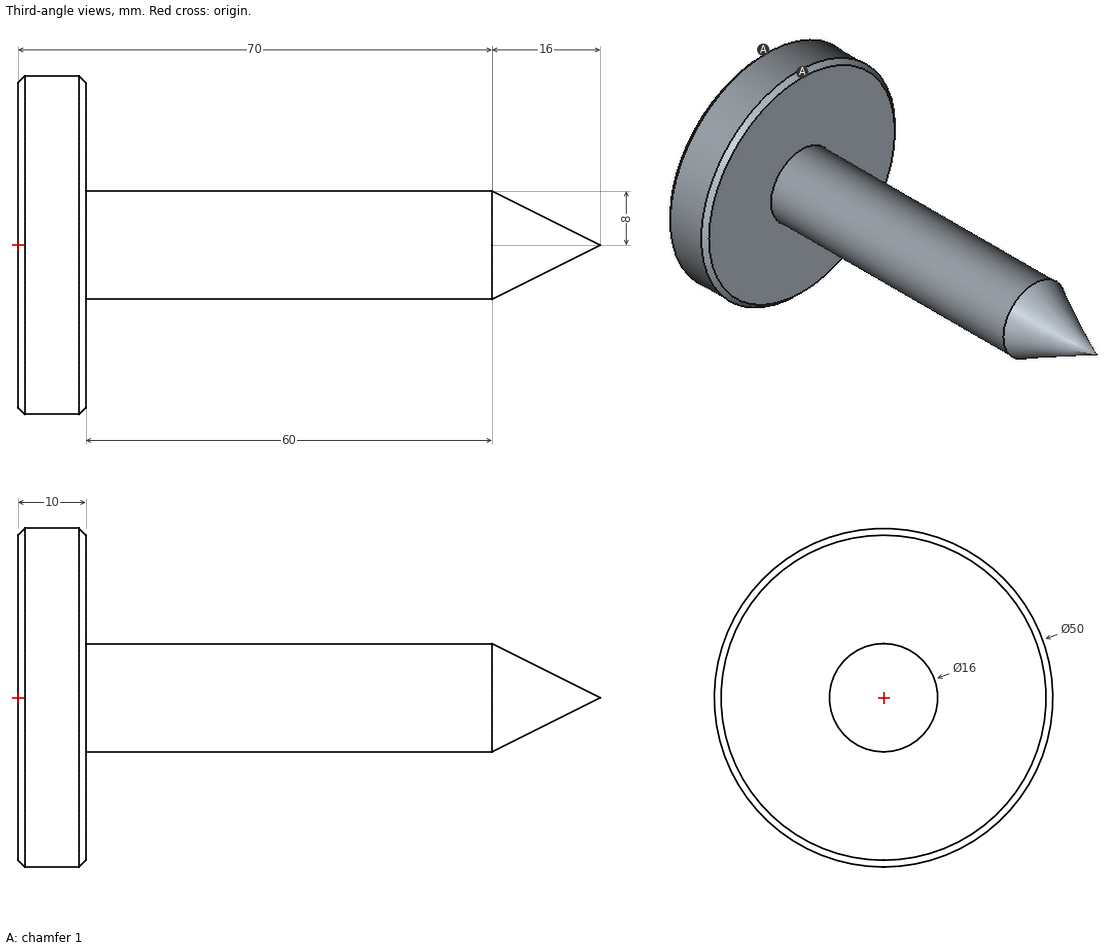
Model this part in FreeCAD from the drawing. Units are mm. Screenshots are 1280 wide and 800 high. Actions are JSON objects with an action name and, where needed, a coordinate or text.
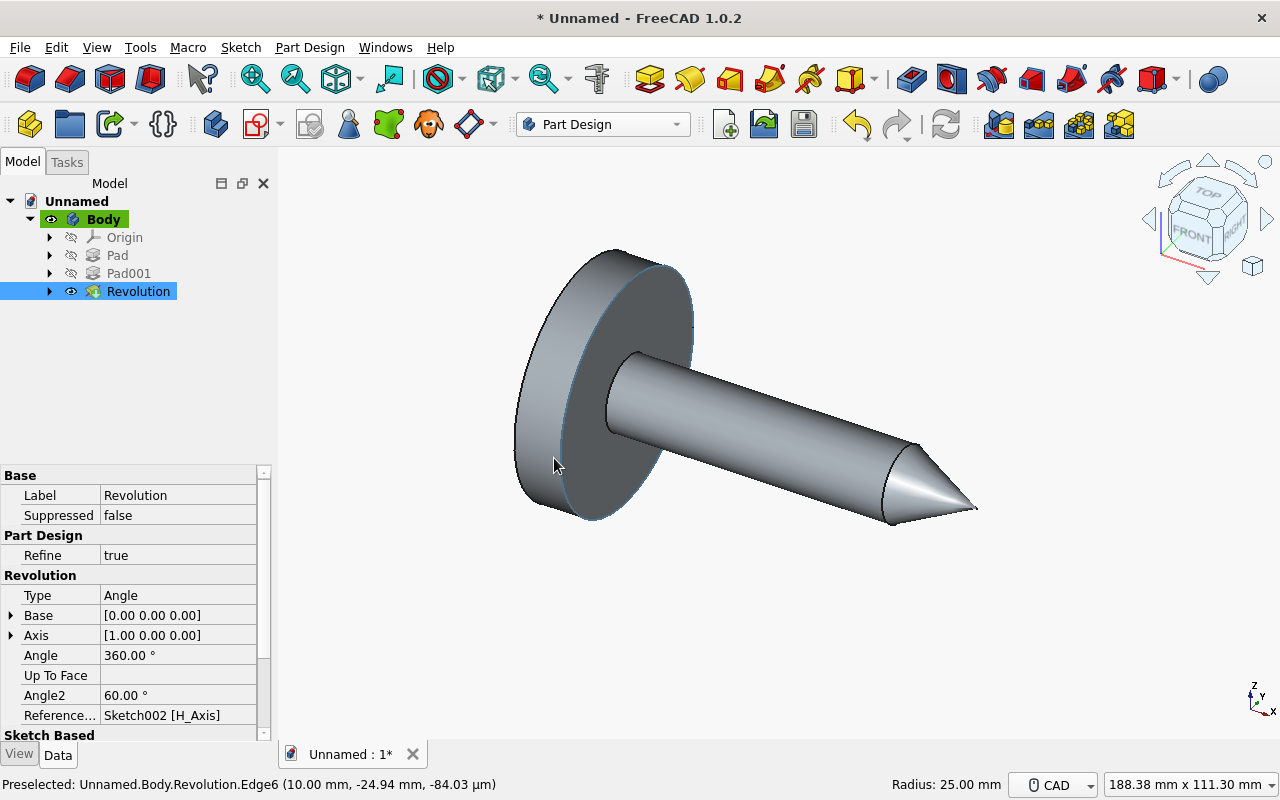
{"action": "key", "text": "0"}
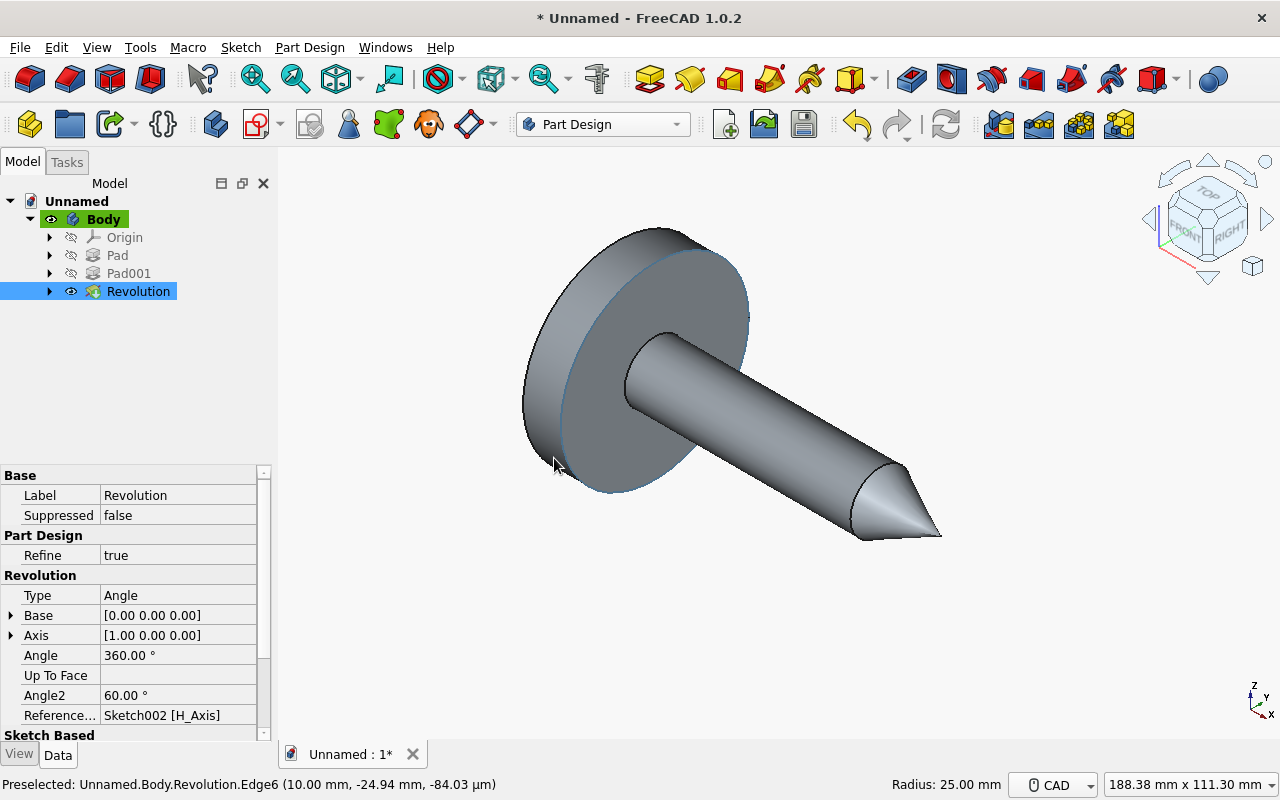
{"action": "key", "text": "2"}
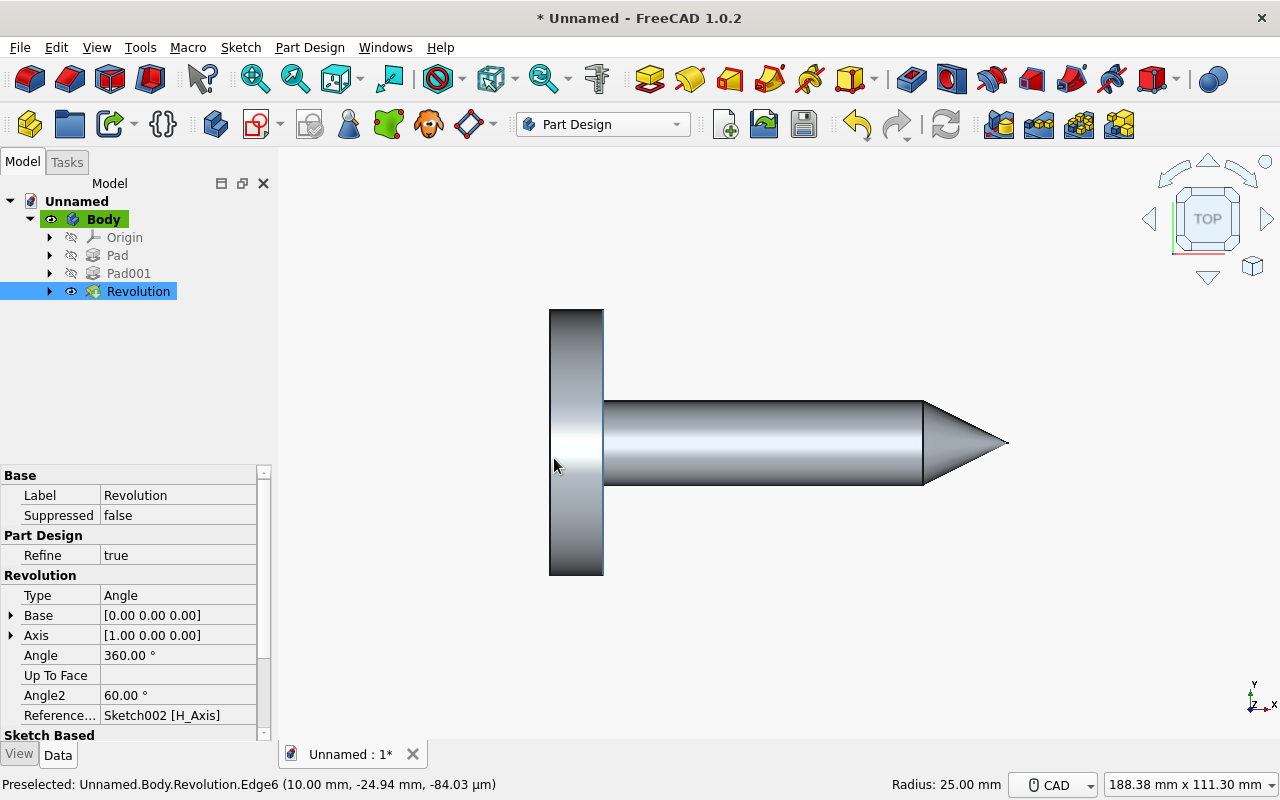
{"action": "left_click", "coordinate": [550, 550], "text": "ctrl"}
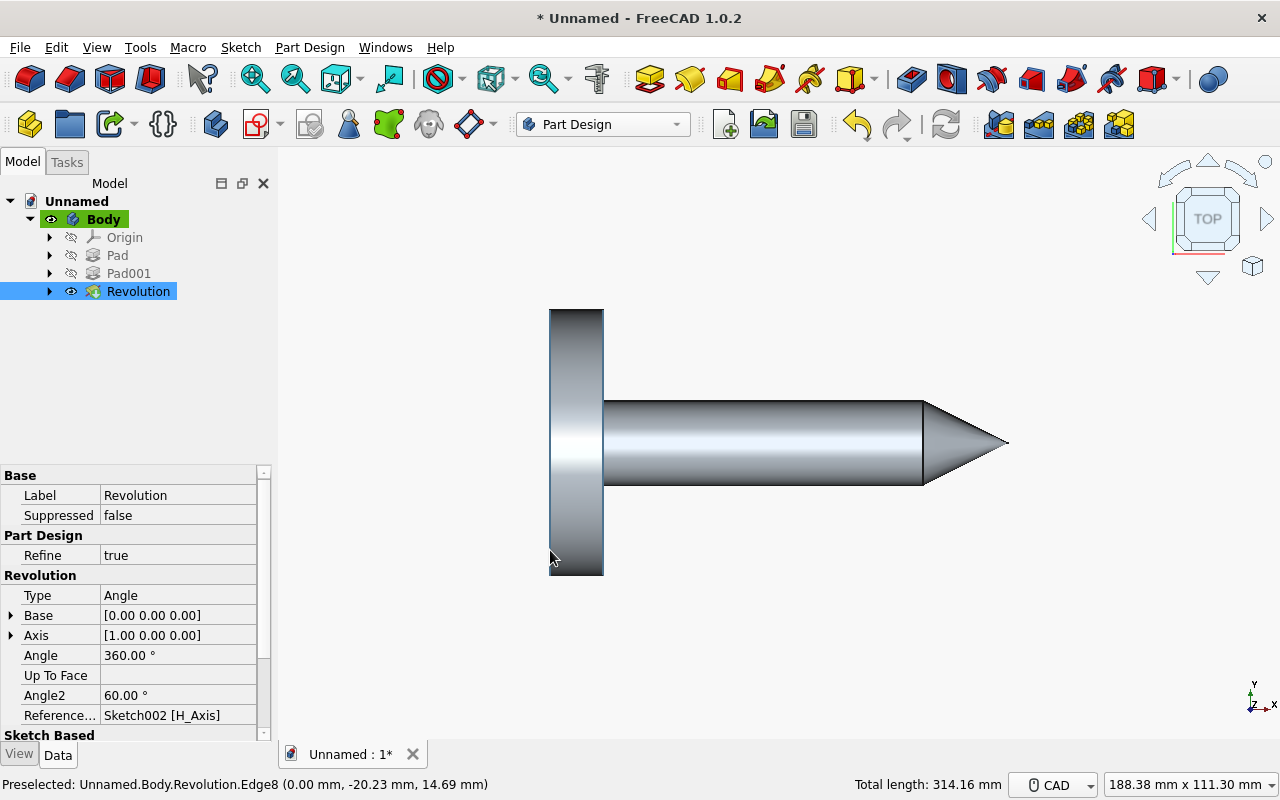
{"action": "left_click", "coordinate": [70, 80]}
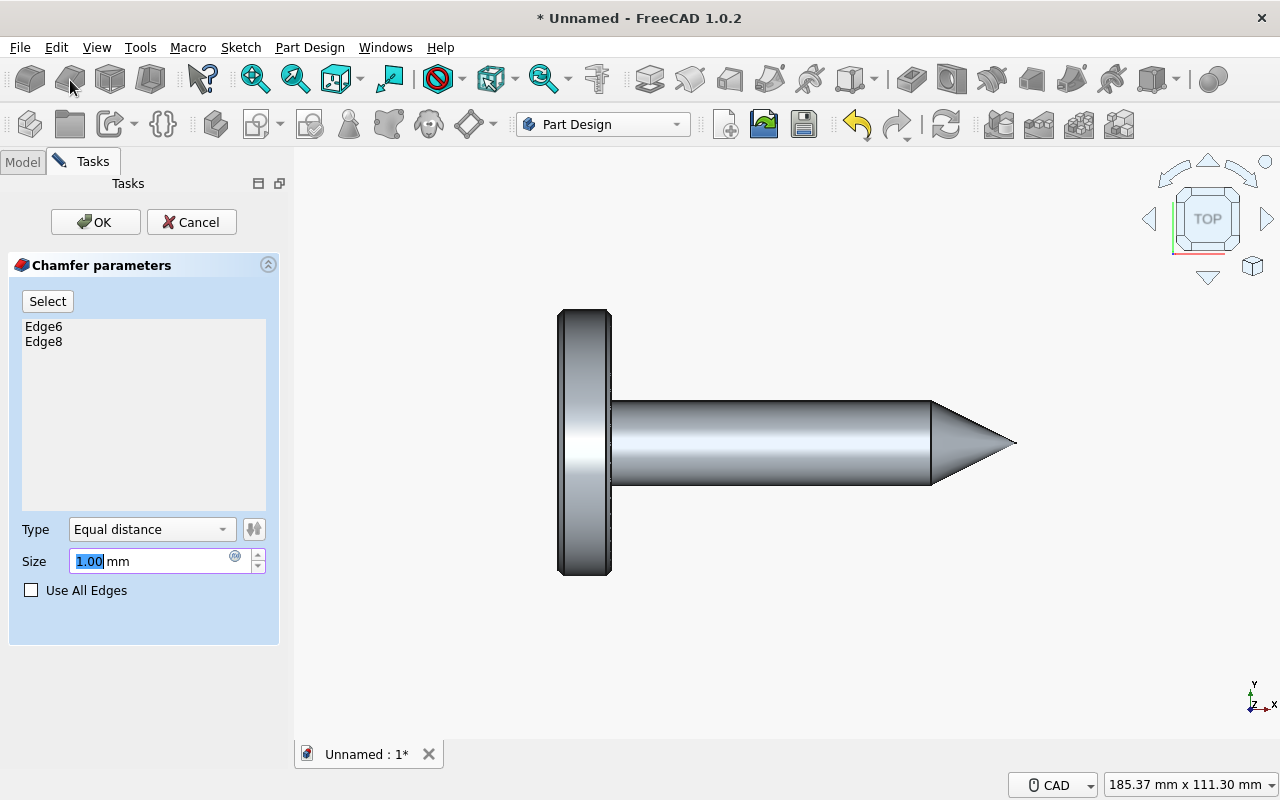
{"action": "type", "text": "1"}
{"action": "key", "text": "Tab"}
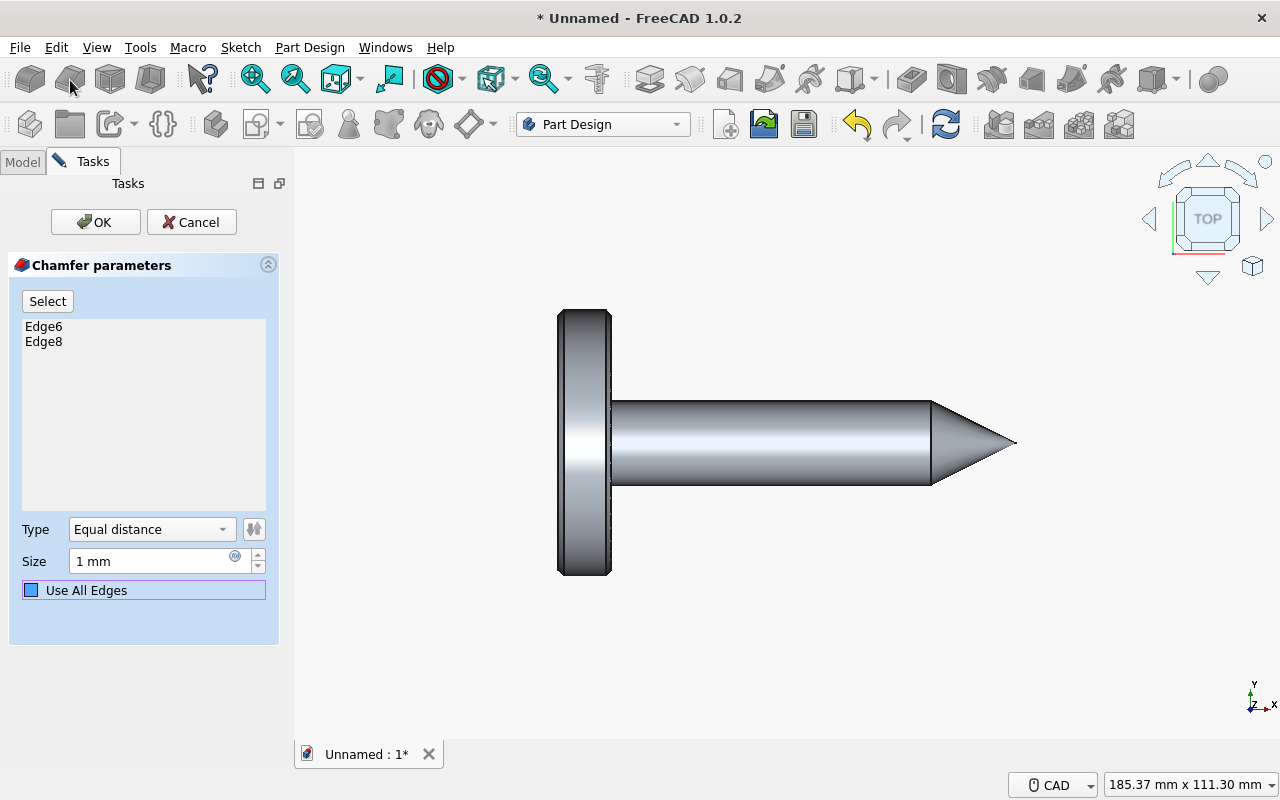
{"action": "left_click", "coordinate": [96, 222]}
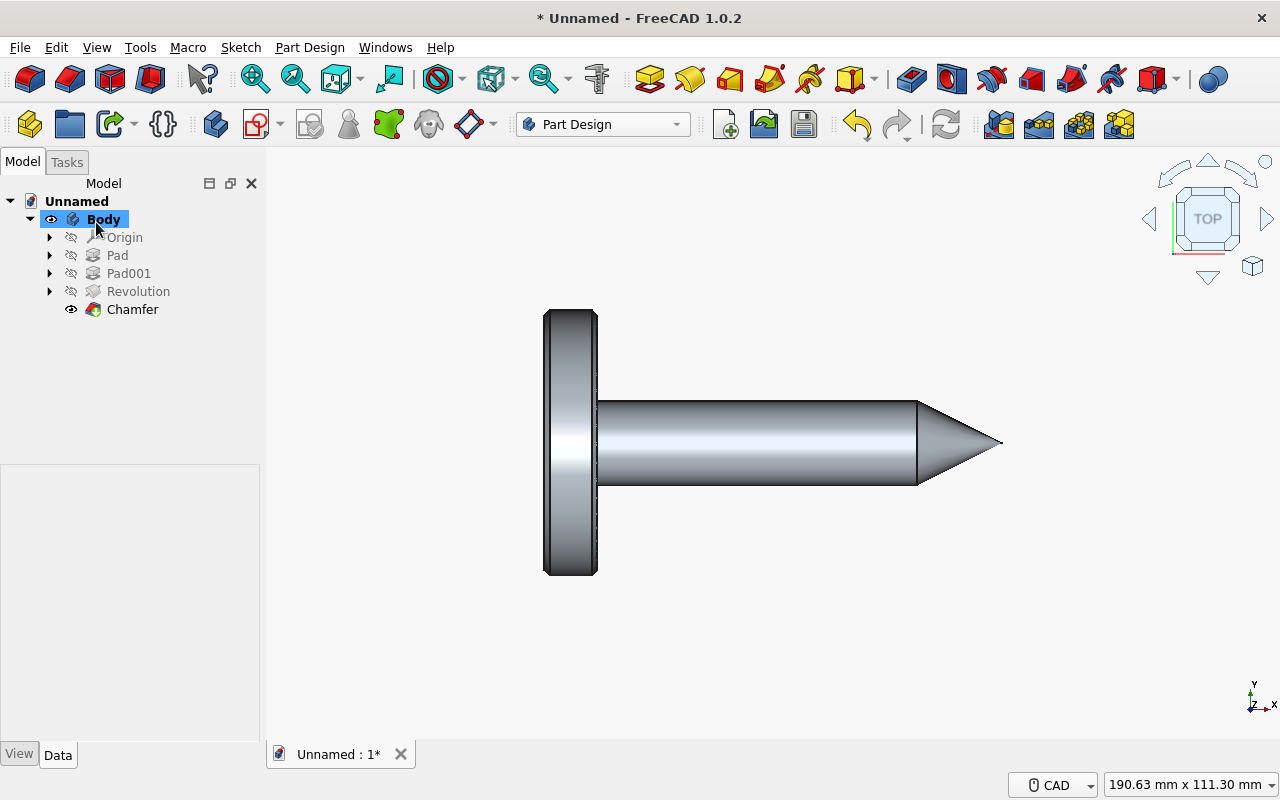
{"action": "key", "text": "0"}